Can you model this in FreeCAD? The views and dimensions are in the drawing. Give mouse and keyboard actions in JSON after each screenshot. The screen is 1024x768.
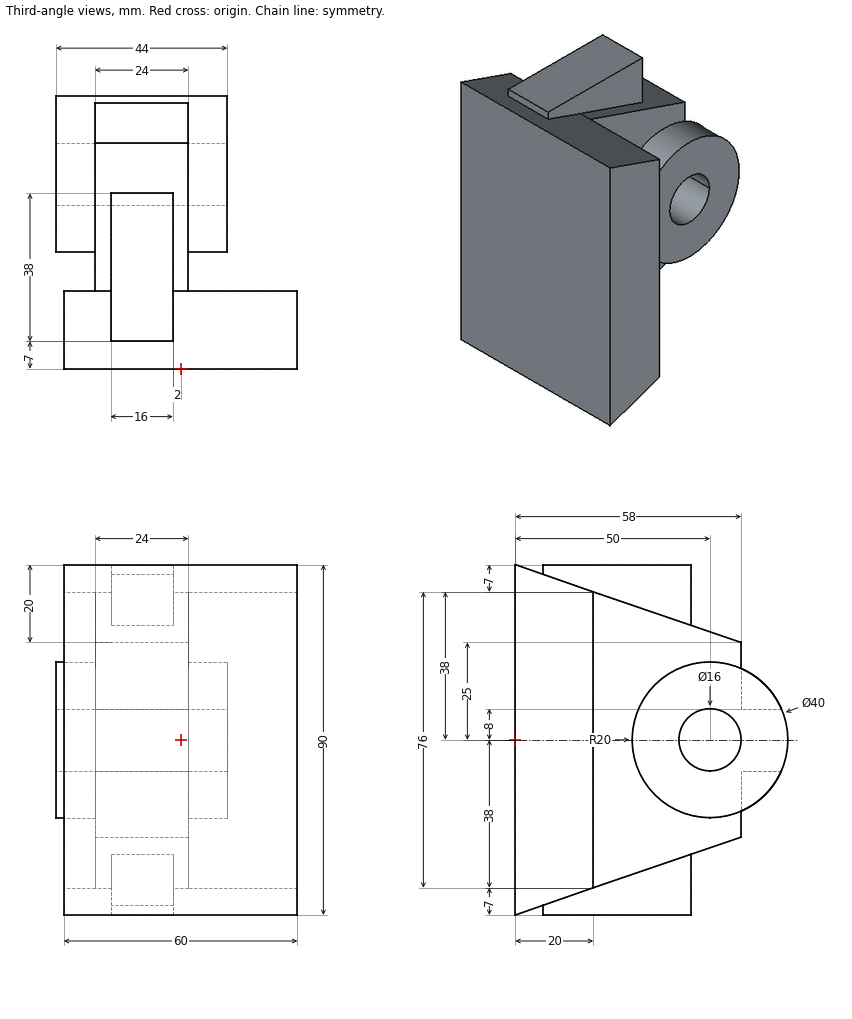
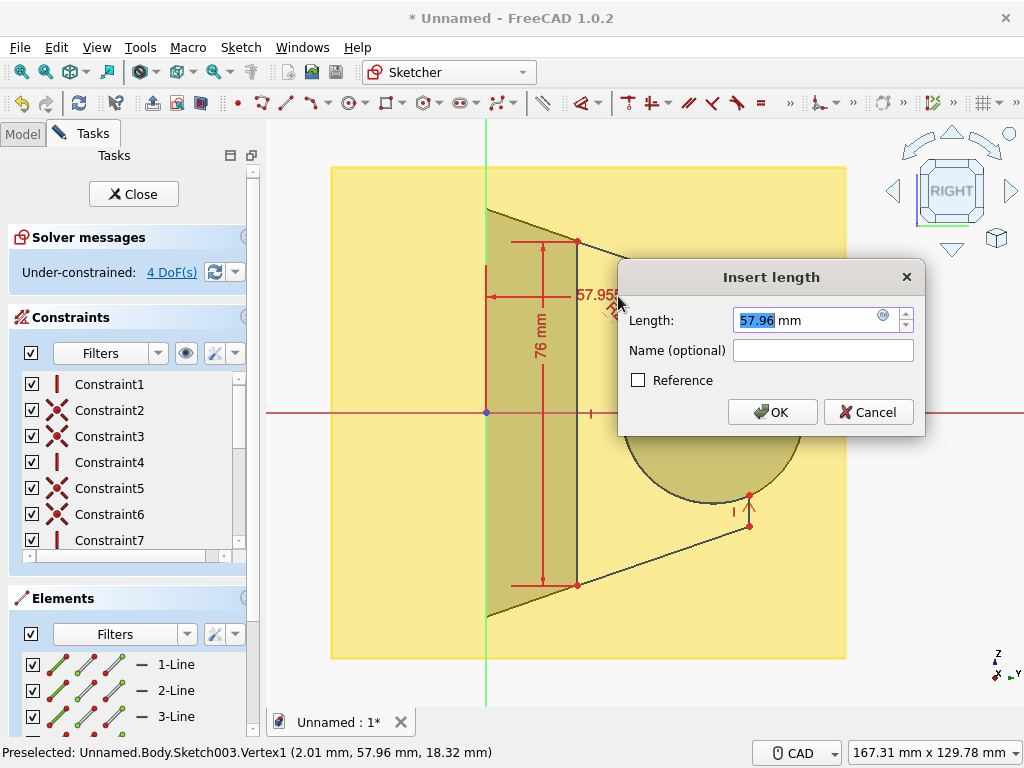
{"action": "type", "text": "58"}
{"action": "key", "text": "Return"}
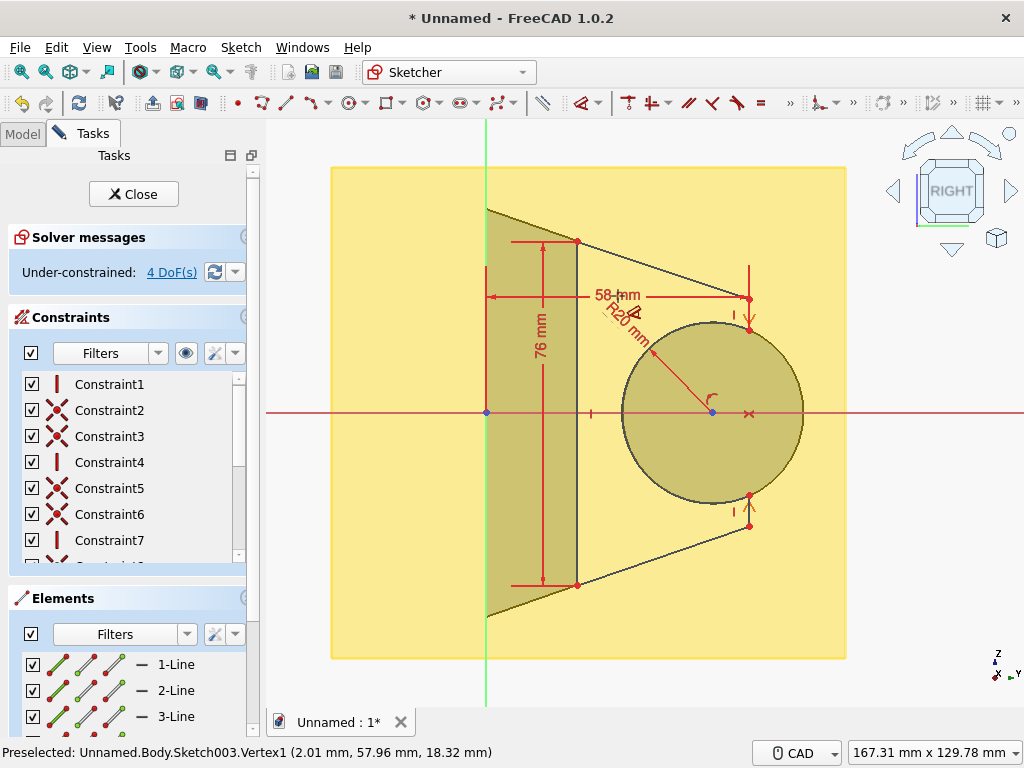
{"action": "left_click", "coordinate": [749, 299]}
{"action": "left_click", "coordinate": [783, 356]}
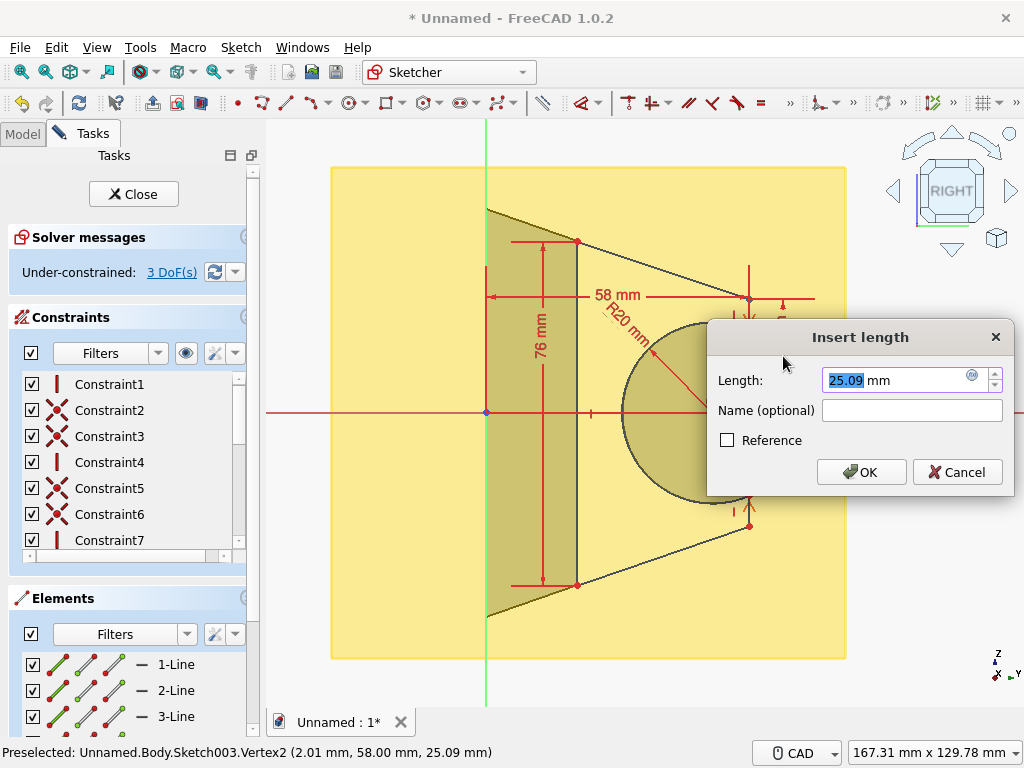
{"action": "type", "text": "25"}
{"action": "key", "text": "Return"}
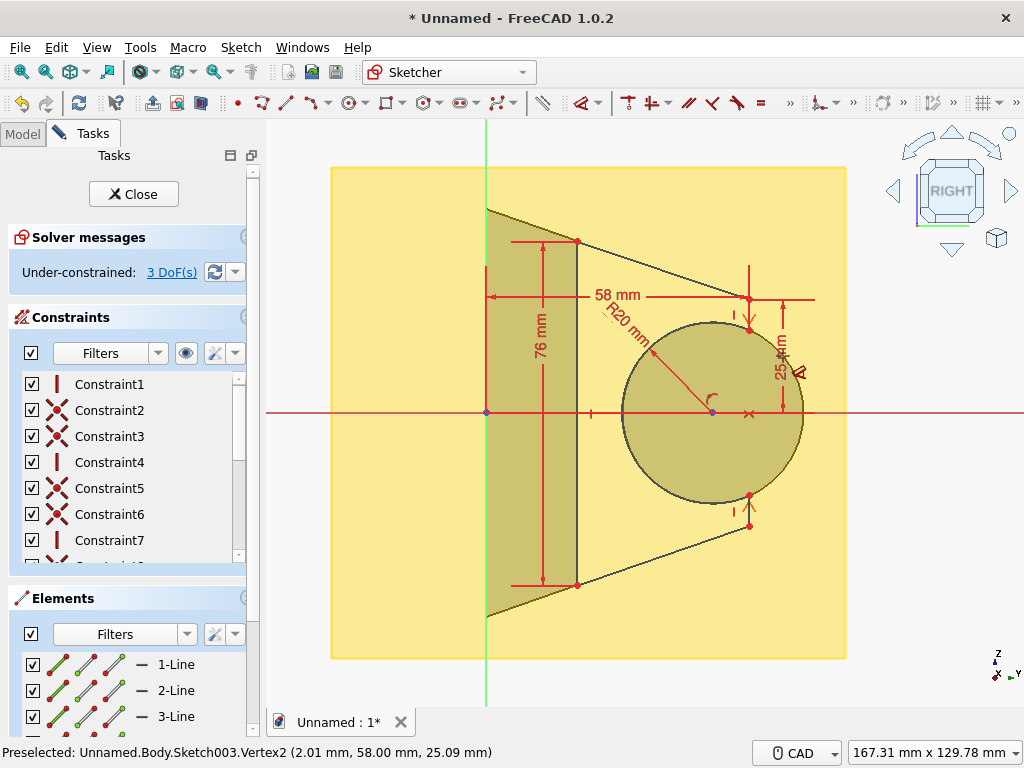
{"action": "left_click", "coordinate": [577, 242]}
{"action": "left_click", "coordinate": [532, 208]}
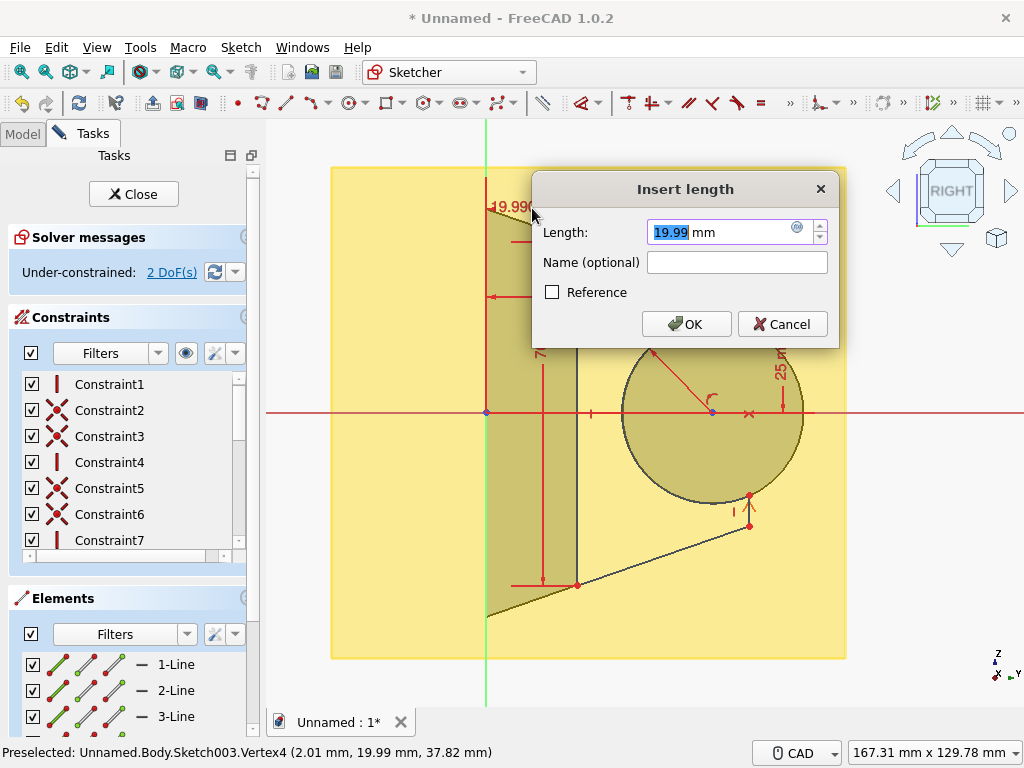
{"action": "type", "text": "20"}
{"action": "key", "text": "Return"}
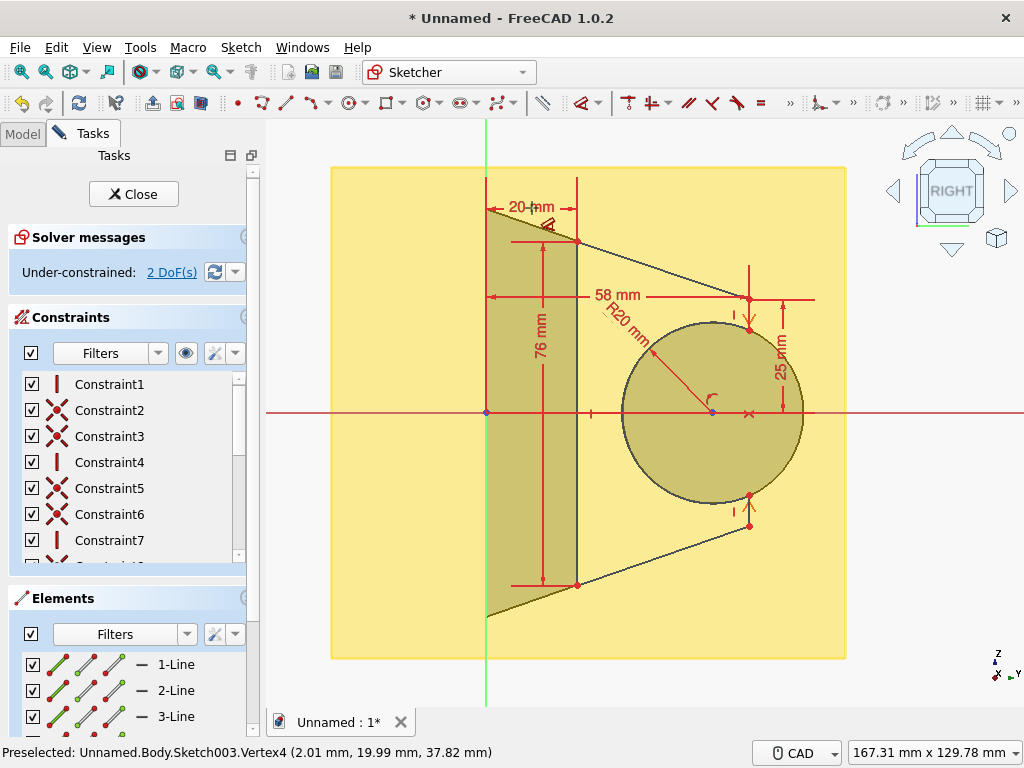
{"action": "left_click", "coordinate": [577, 242]}
{"action": "left_click", "coordinate": [452, 327]}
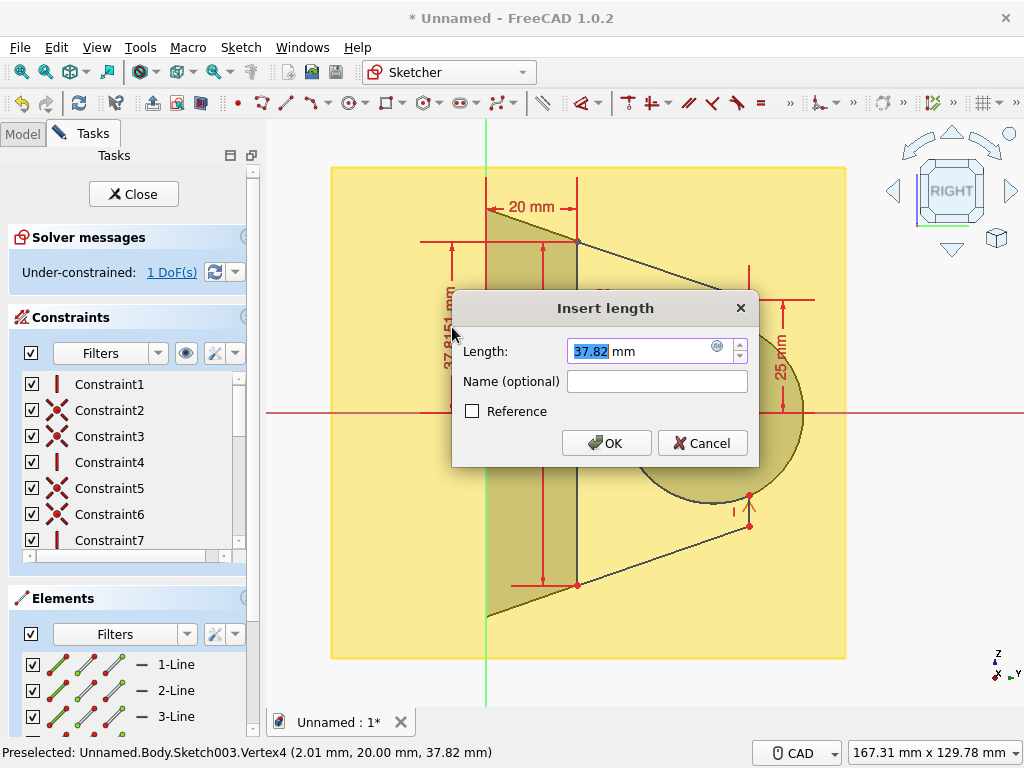
{"action": "type", "text": "38"}
{"action": "key", "text": "Return"}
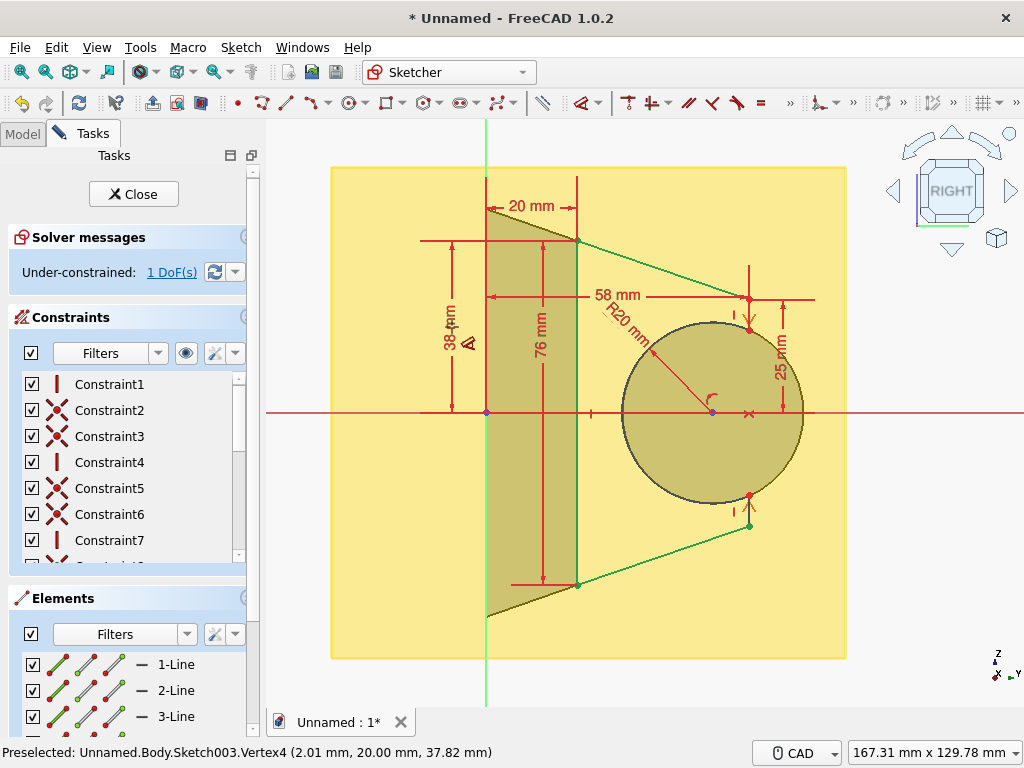
{"action": "left_click", "coordinate": [713, 413]}
{"action": "left_click", "coordinate": [600, 447]}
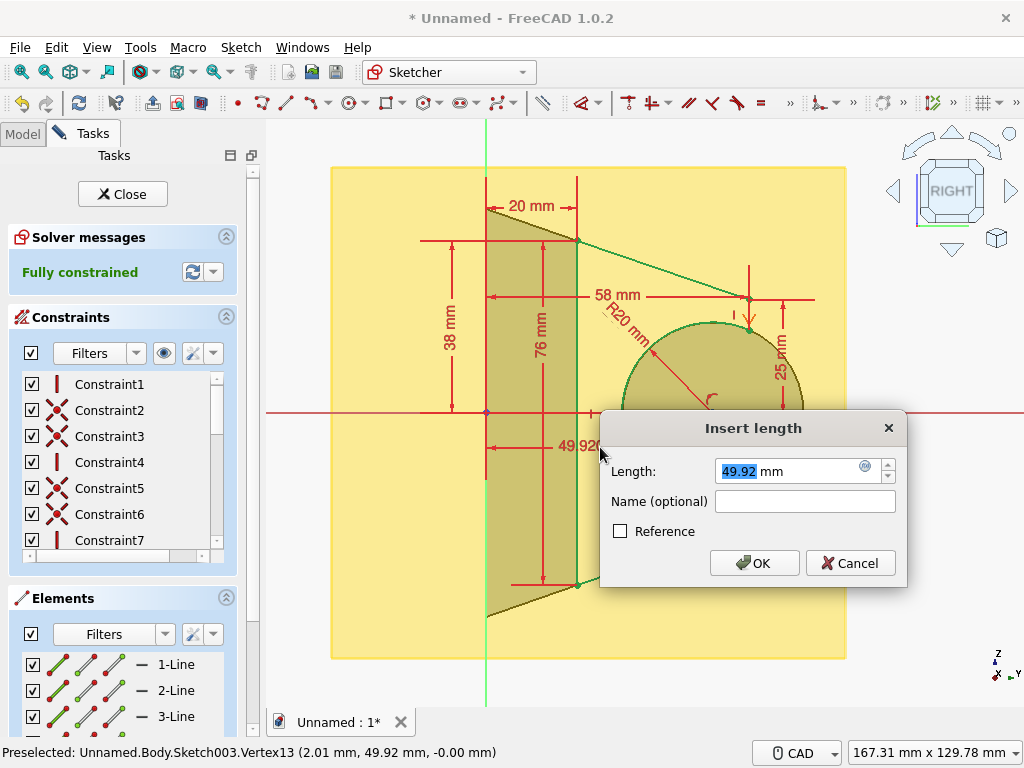
{"action": "type", "text": "50"}
{"action": "key", "text": "Return"}
{"action": "key", "text": "Escape"}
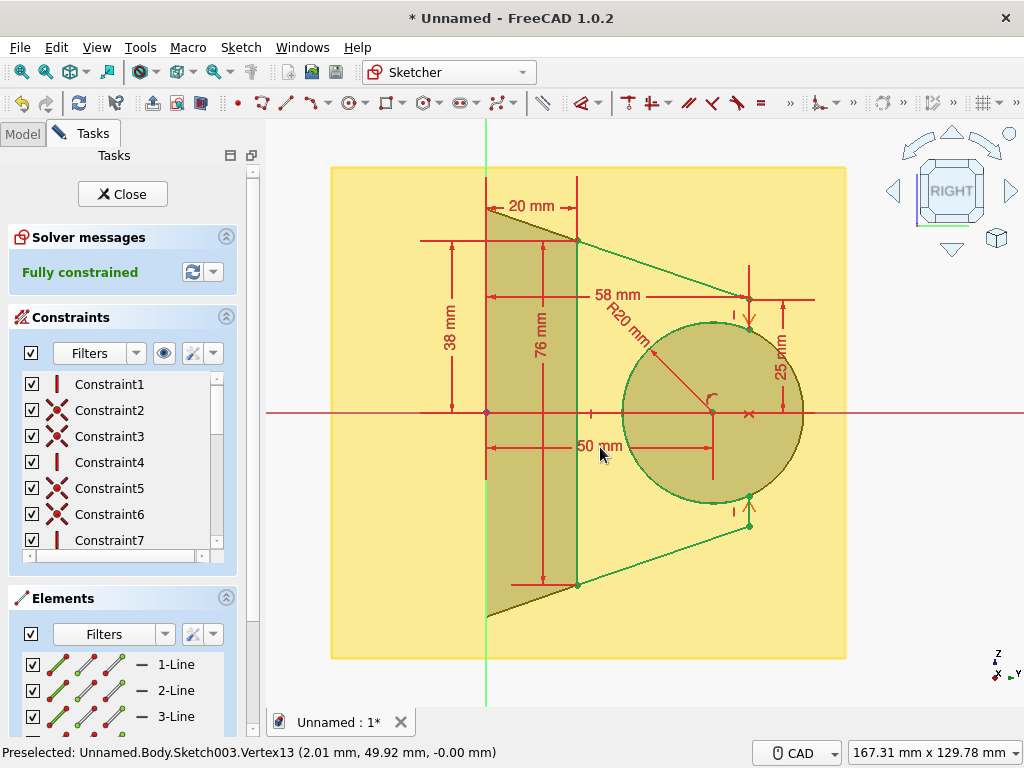
{"action": "left_click", "coordinate": [123, 194]}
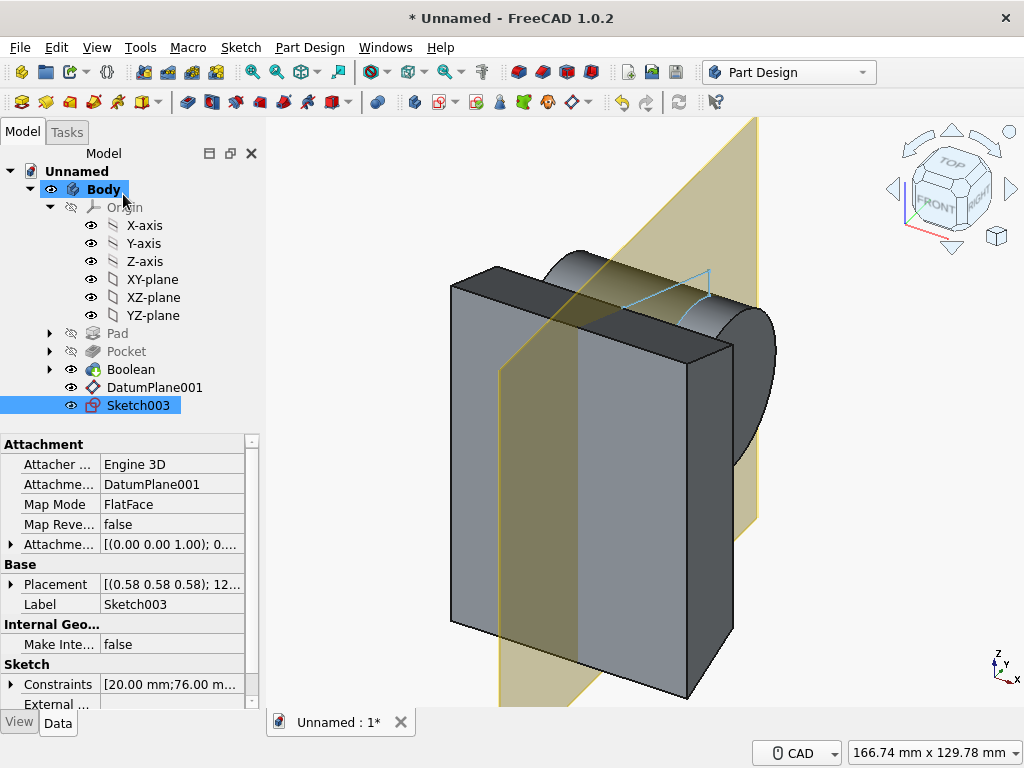
{"action": "left_click", "coordinate": [22, 102]}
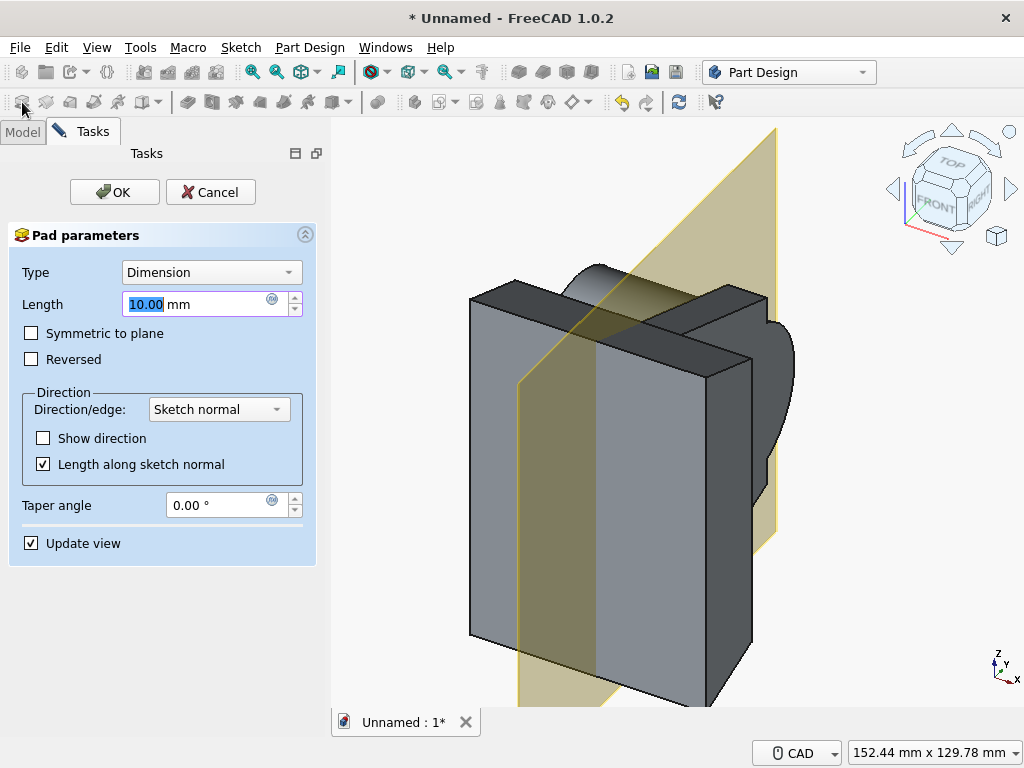
{"action": "type", "text": "24"}
{"action": "key", "text": "Tab"}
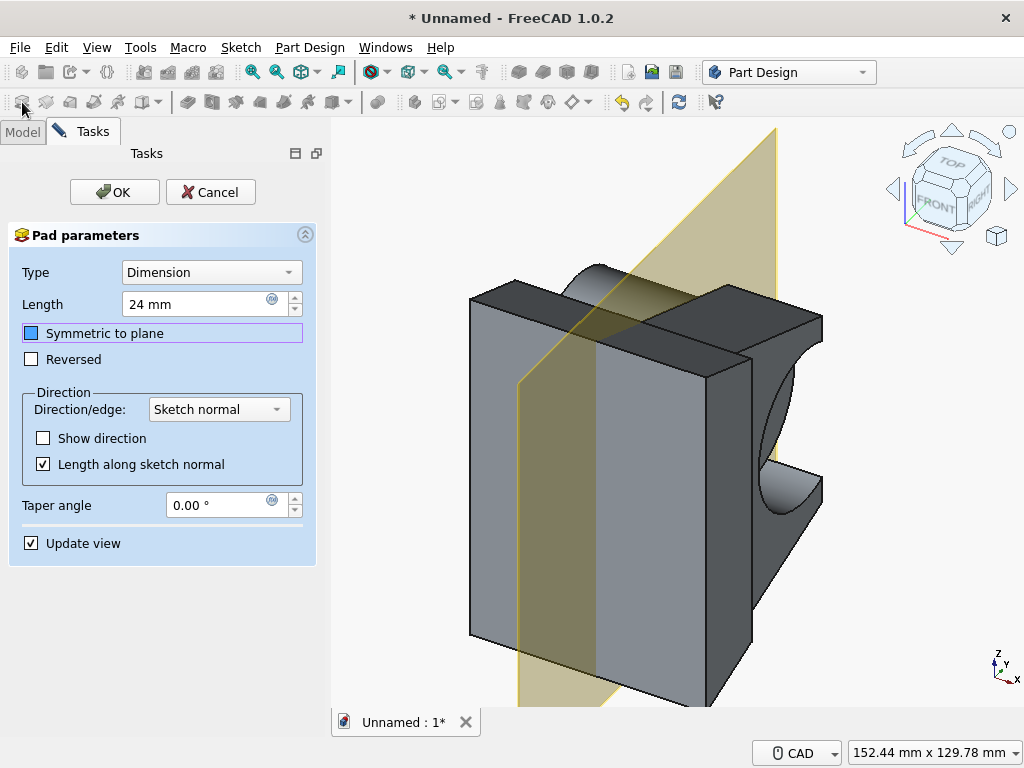
{"action": "left_click", "coordinate": [30, 359]}